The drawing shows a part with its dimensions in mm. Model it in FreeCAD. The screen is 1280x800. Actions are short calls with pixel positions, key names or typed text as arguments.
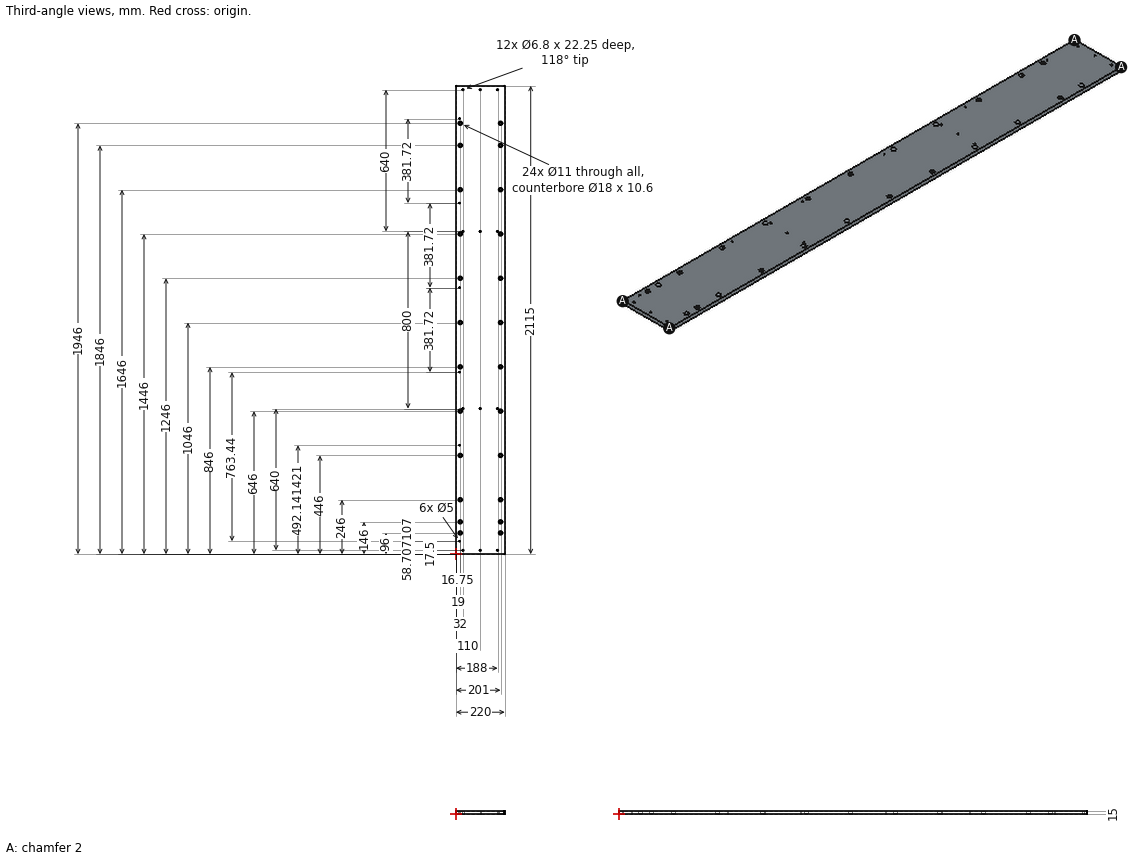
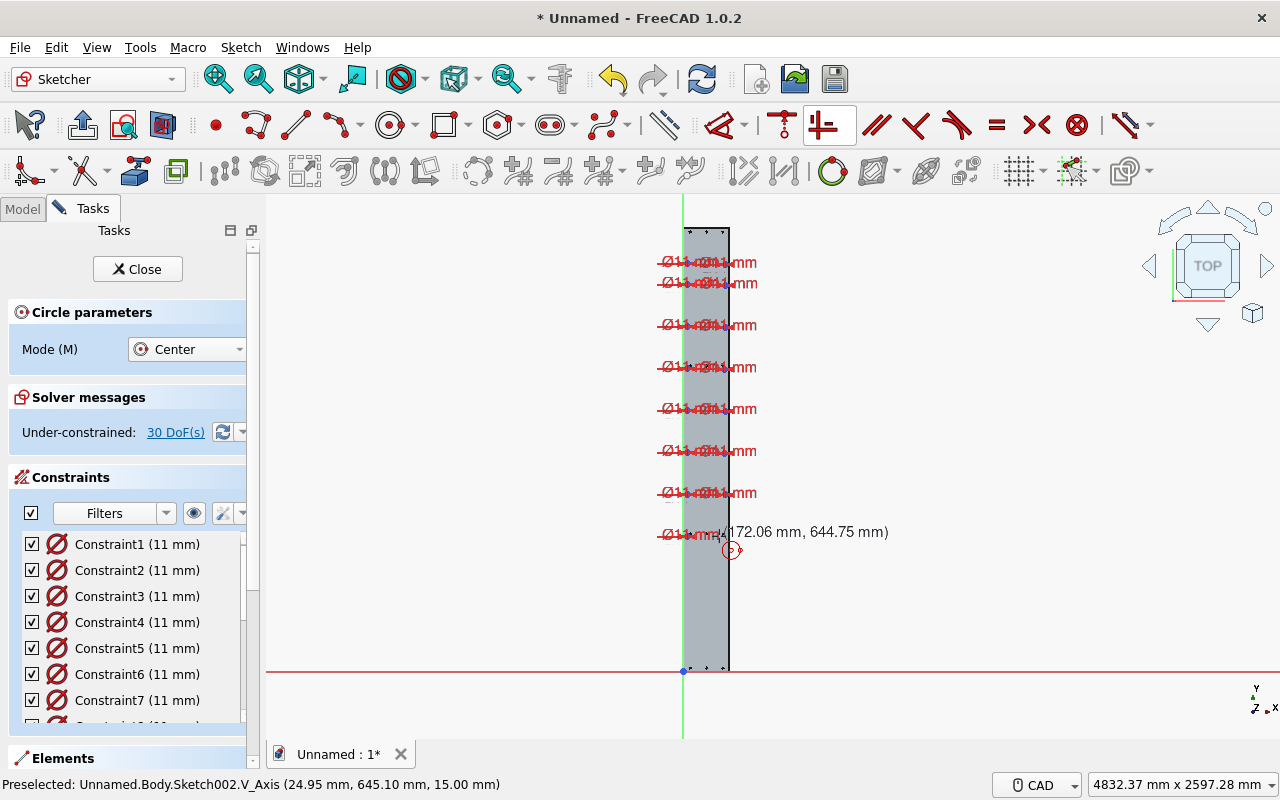
click(725, 536)
move(726, 536)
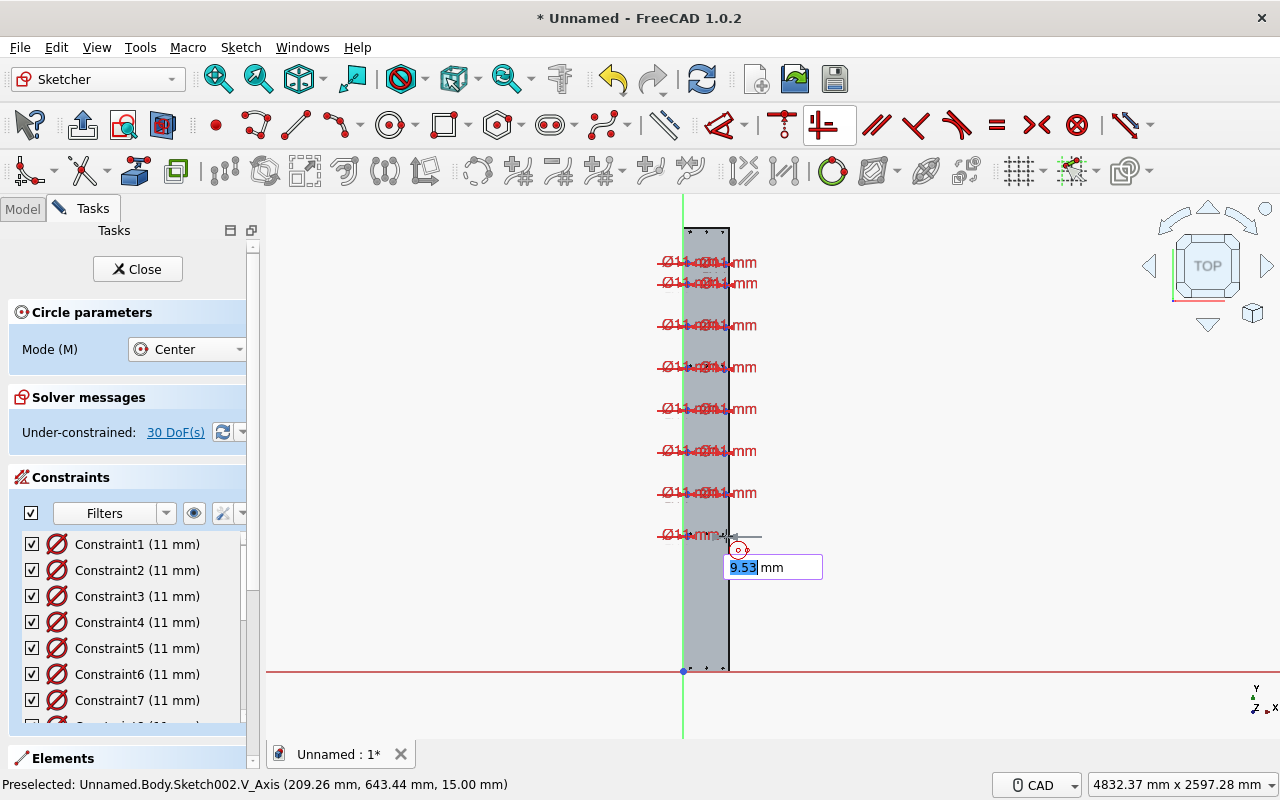
text(11)
key(Return)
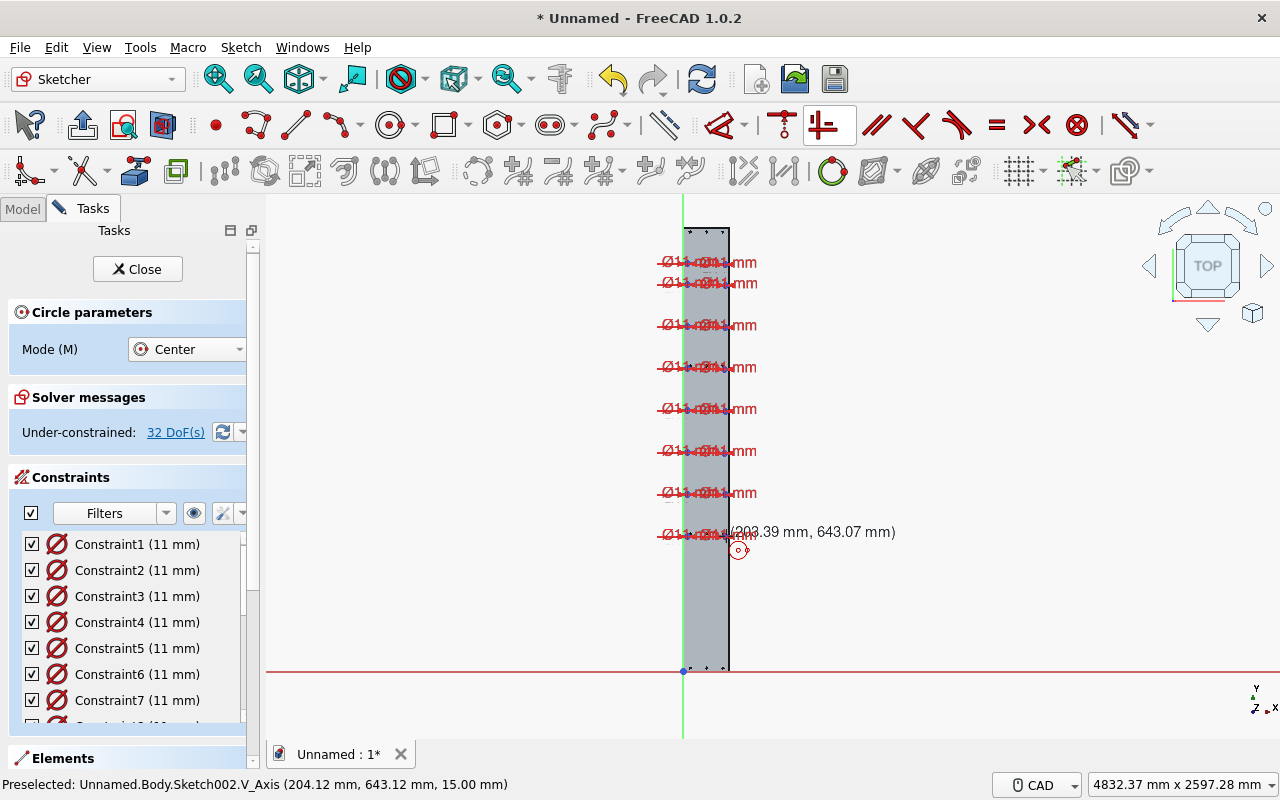
scroll(687, 578, up, 15)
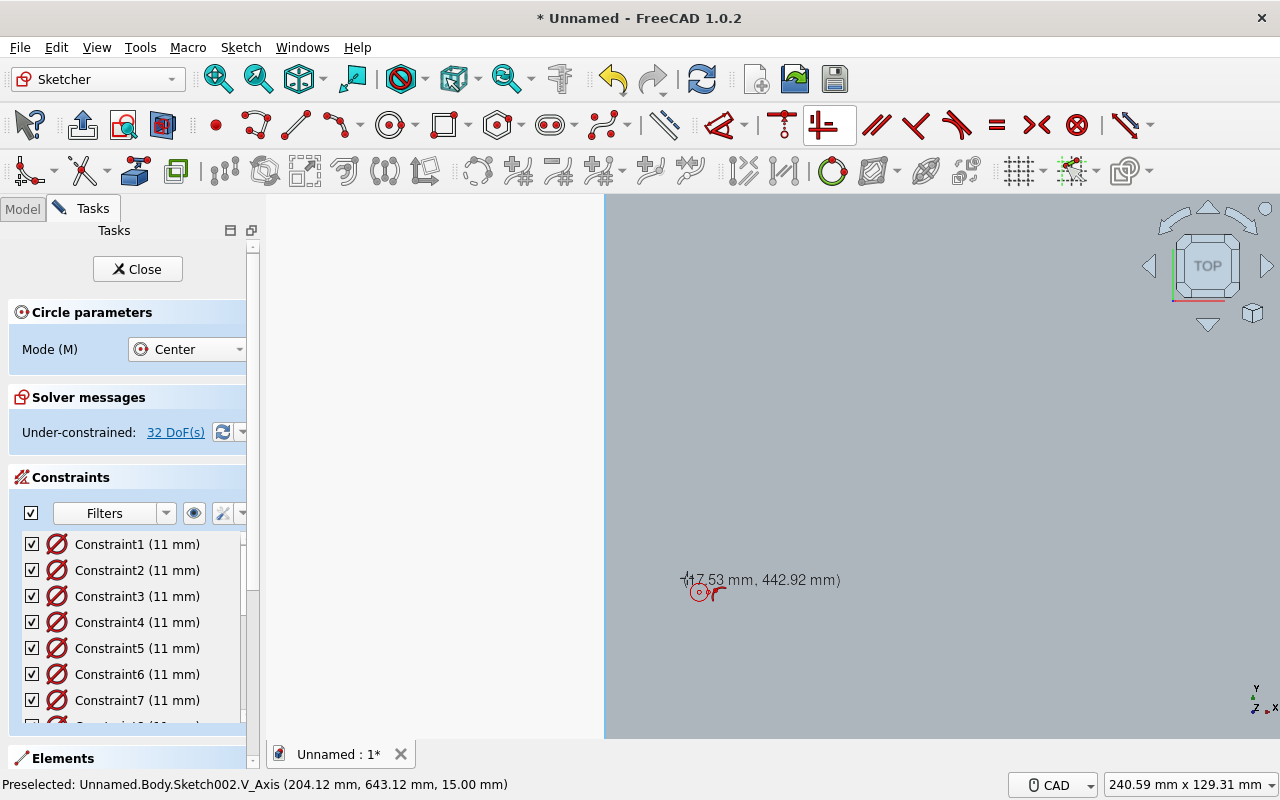
scroll(687, 578, down, 15)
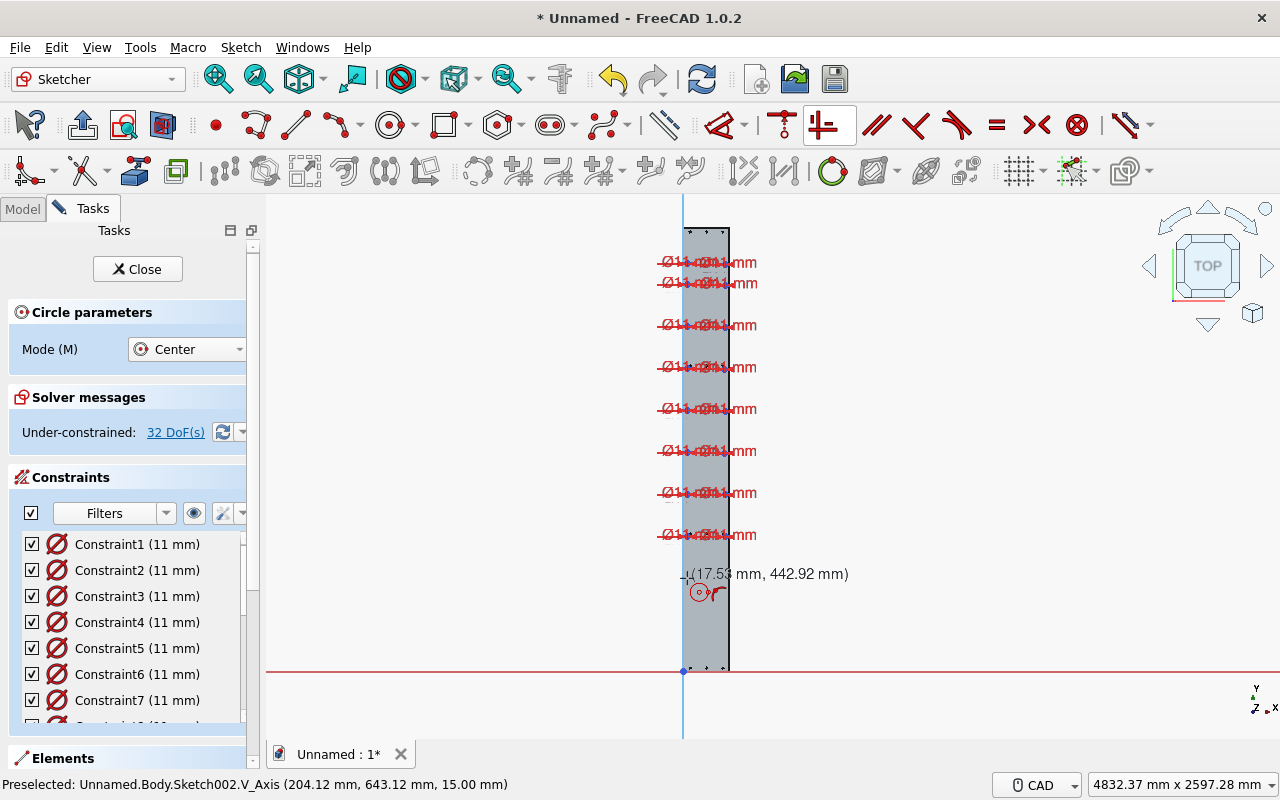
scroll(687, 578, up, 7)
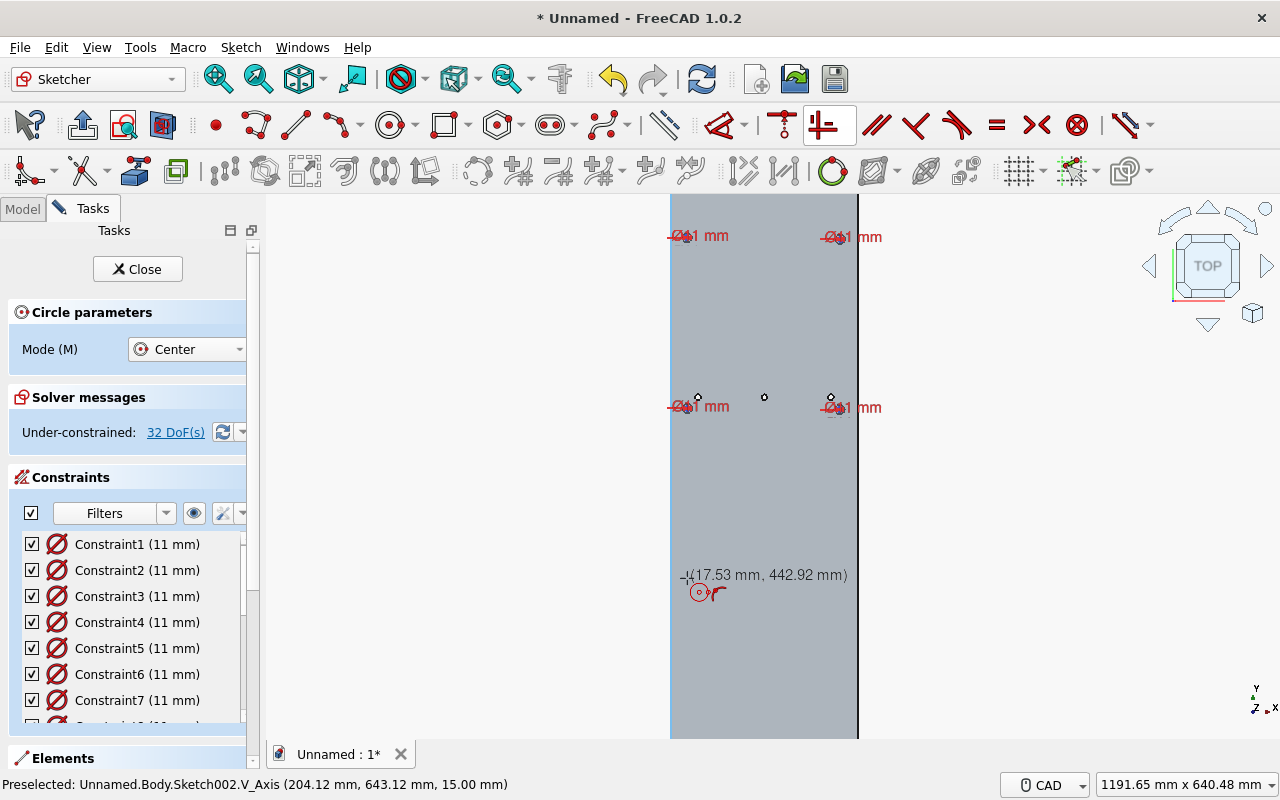
click(687, 577)
move(690, 574)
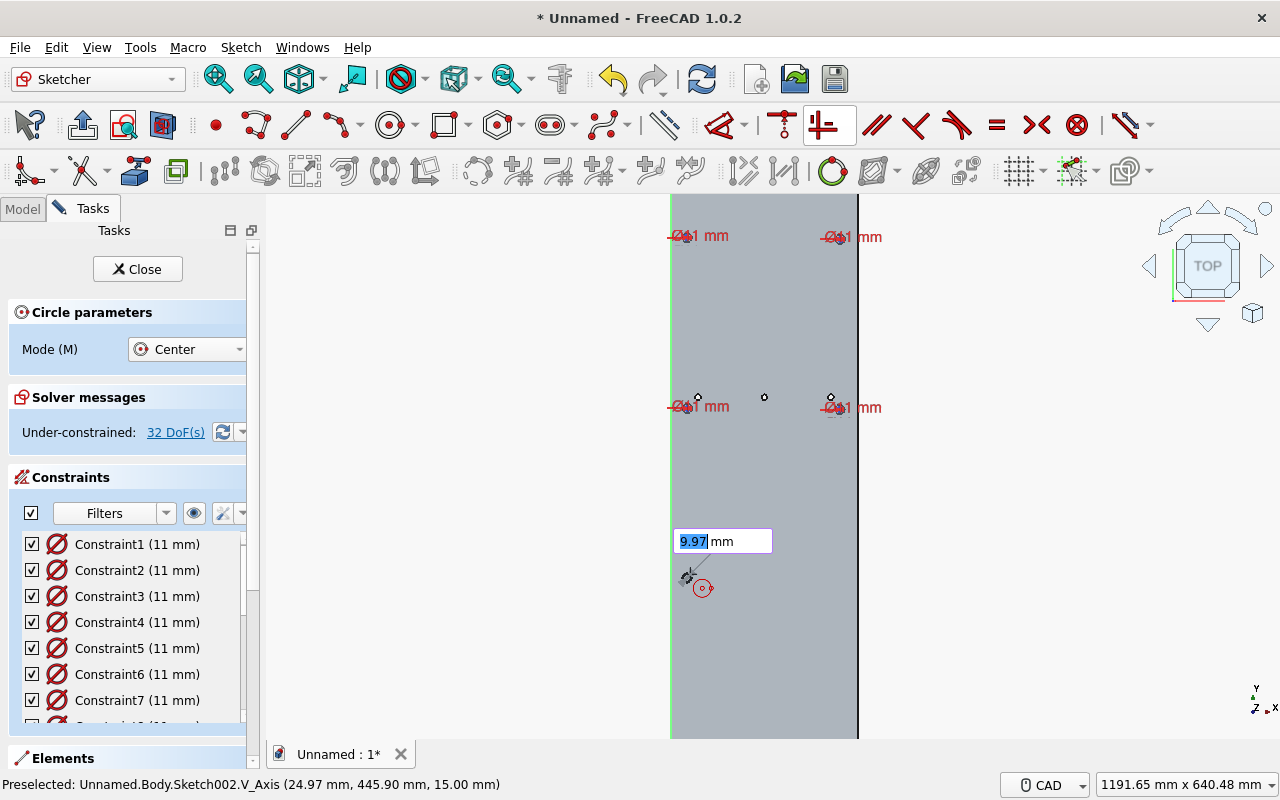
text(11)
key(Return)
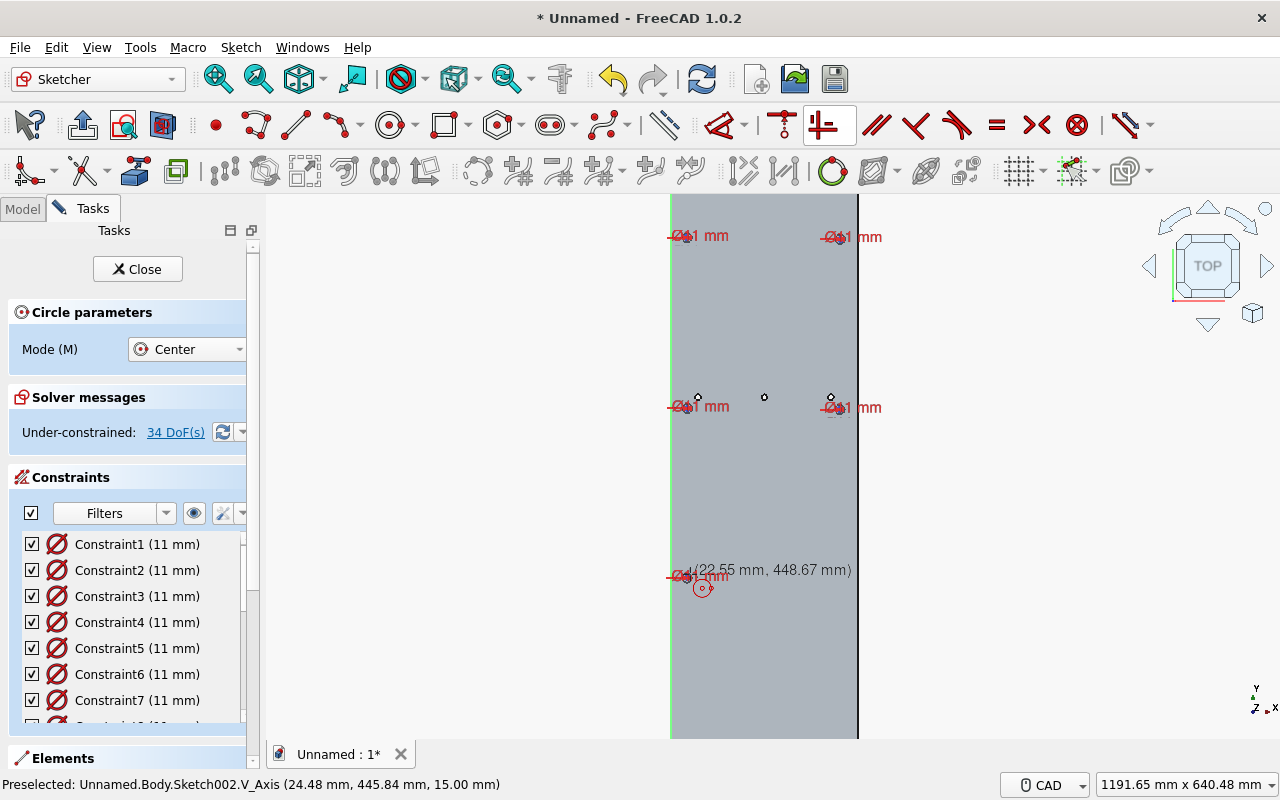
scroll(842, 577, up, 8)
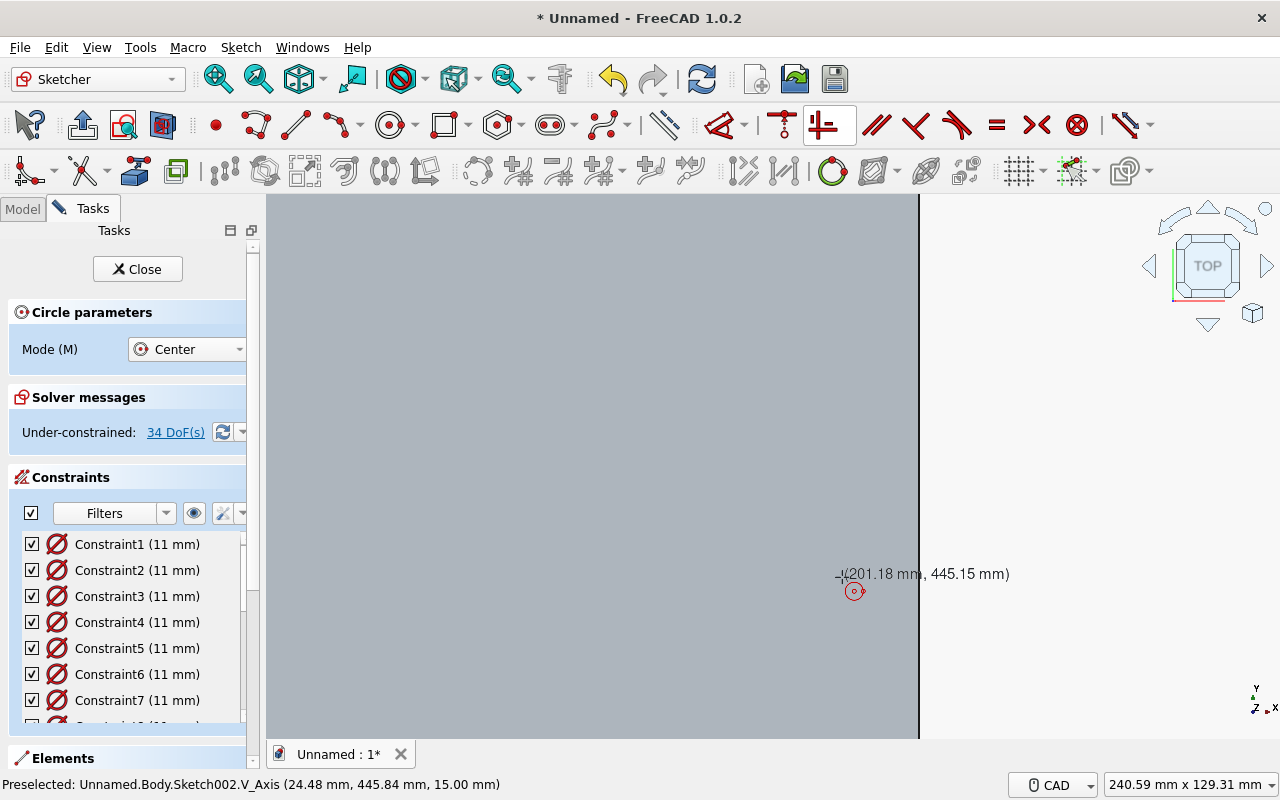
scroll(719, 578, down, 15)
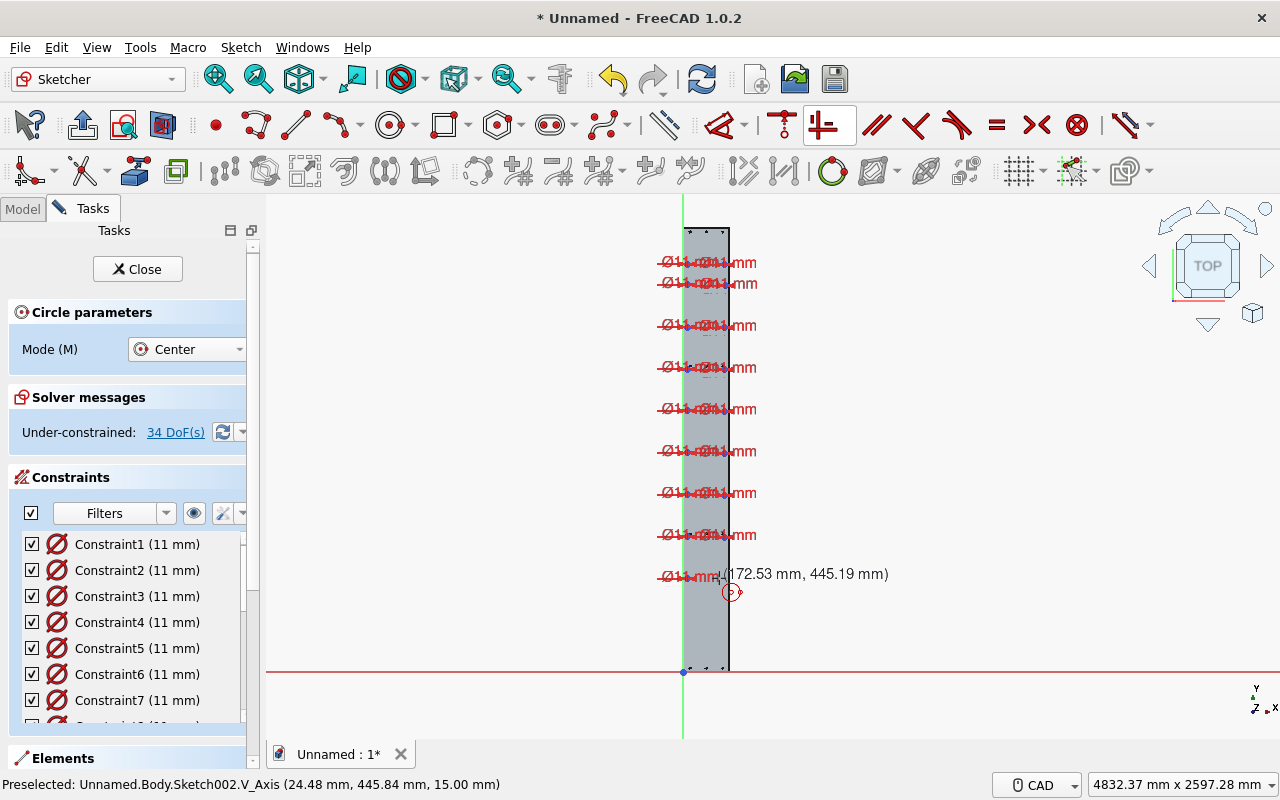
click(725, 579)
move(726, 578)